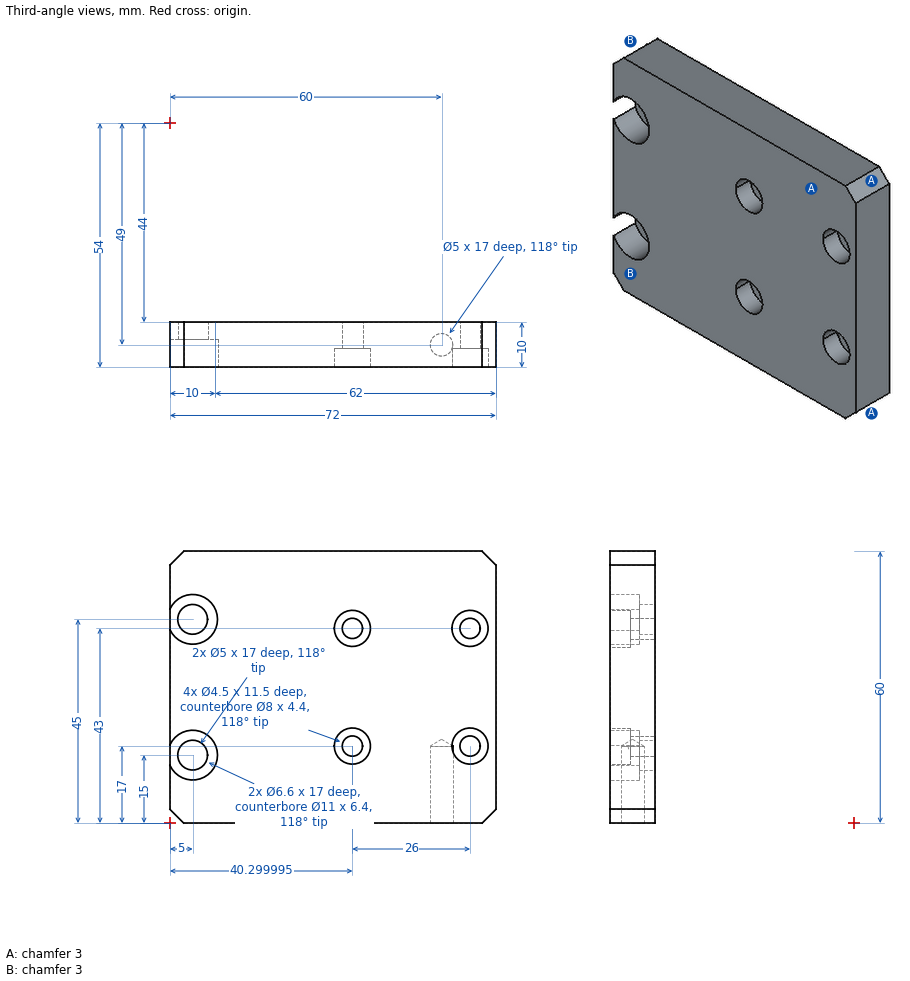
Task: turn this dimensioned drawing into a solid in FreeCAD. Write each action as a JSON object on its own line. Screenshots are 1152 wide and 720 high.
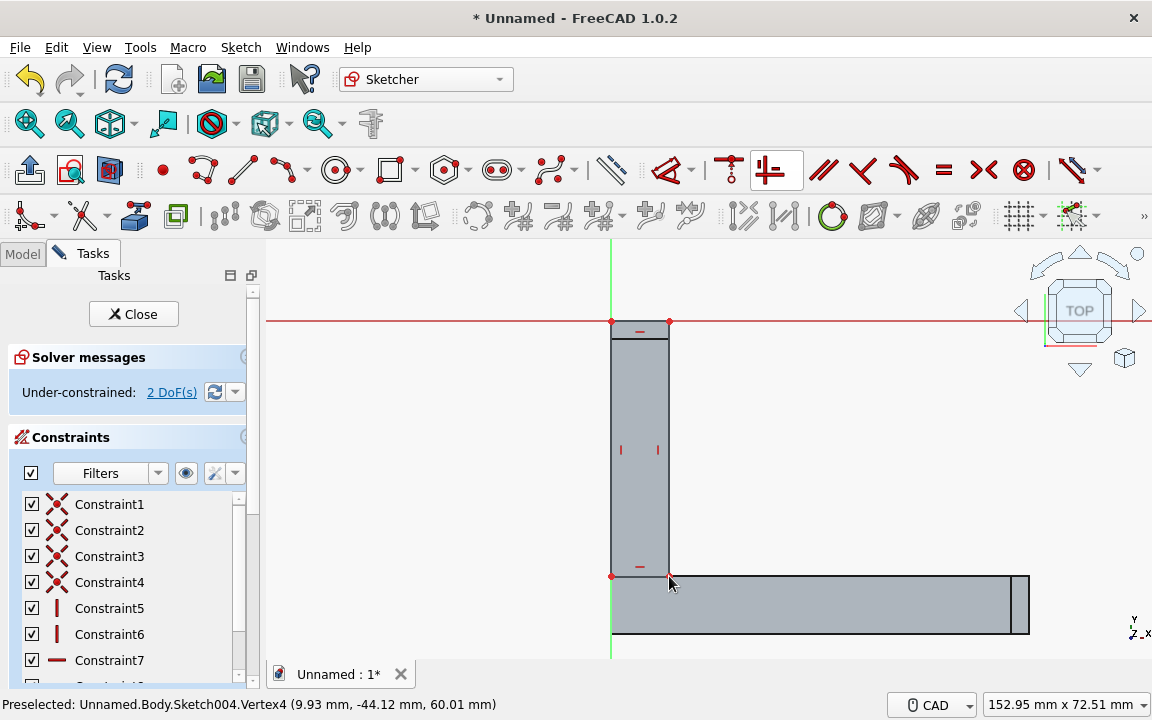
{"action": "left_click", "coordinate": [666, 170]}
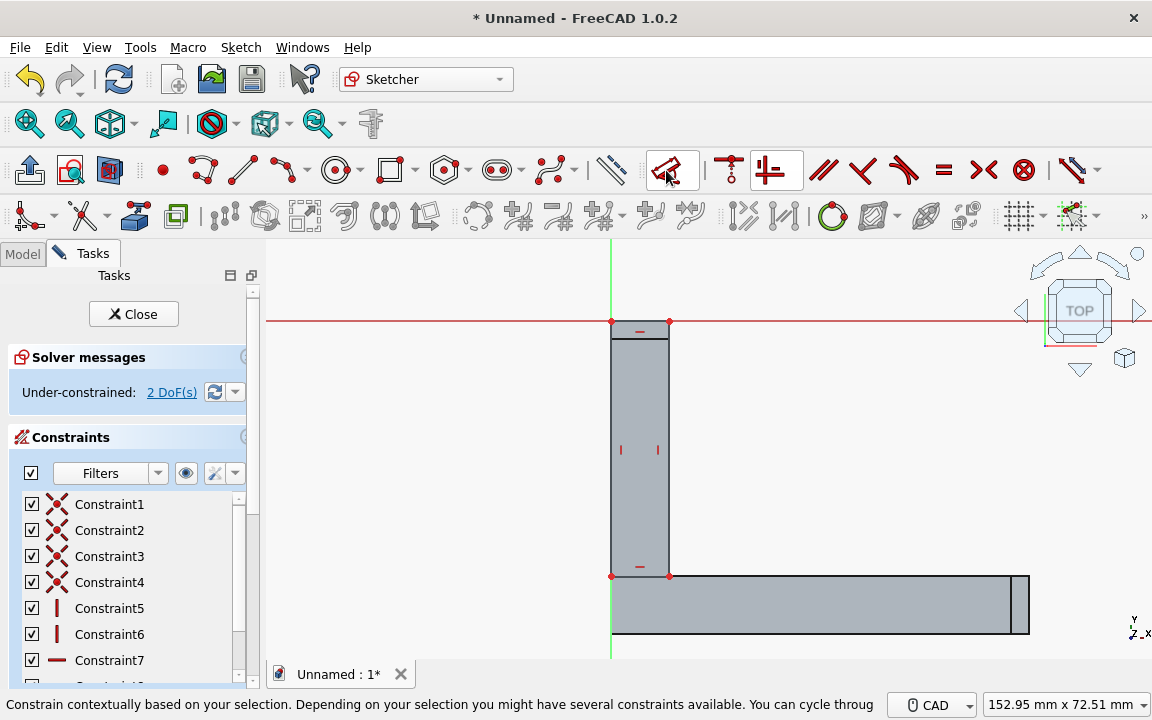
{"action": "left_click", "coordinate": [611, 398]}
{"action": "left_click", "coordinate": [577, 449]}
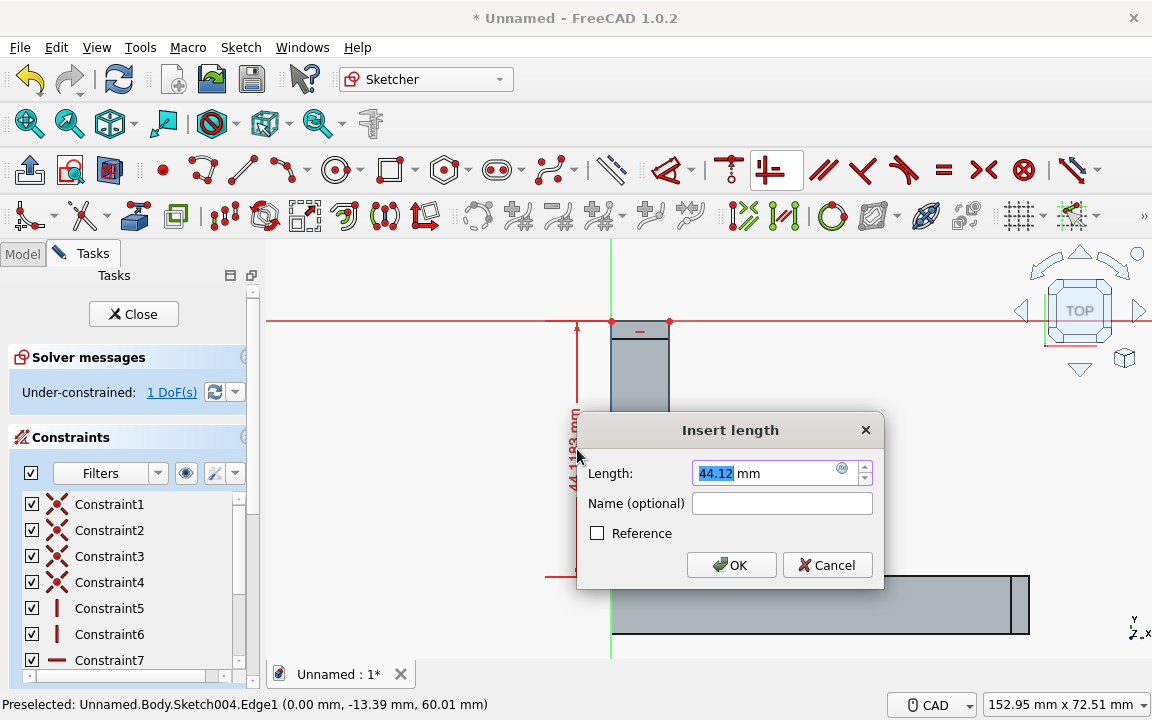
{"action": "type", "text": "44"}
{"action": "key", "text": "Return"}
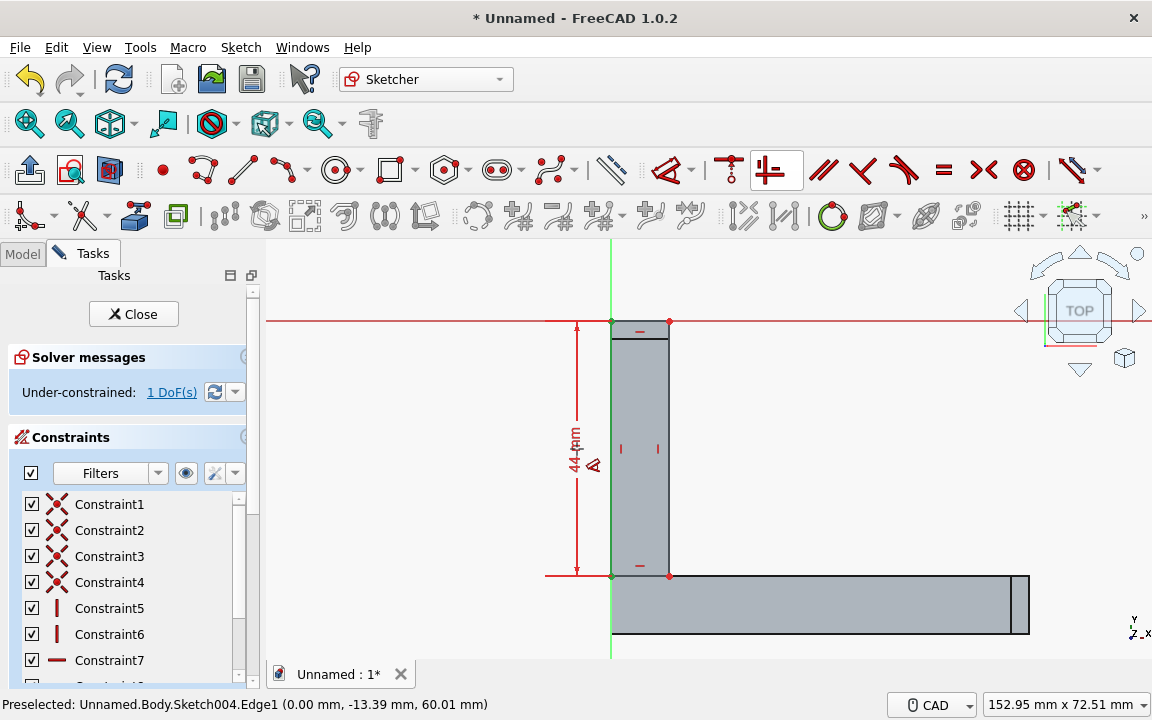
{"action": "left_click", "coordinate": [629, 576]}
{"action": "left_click", "coordinate": [640, 610]}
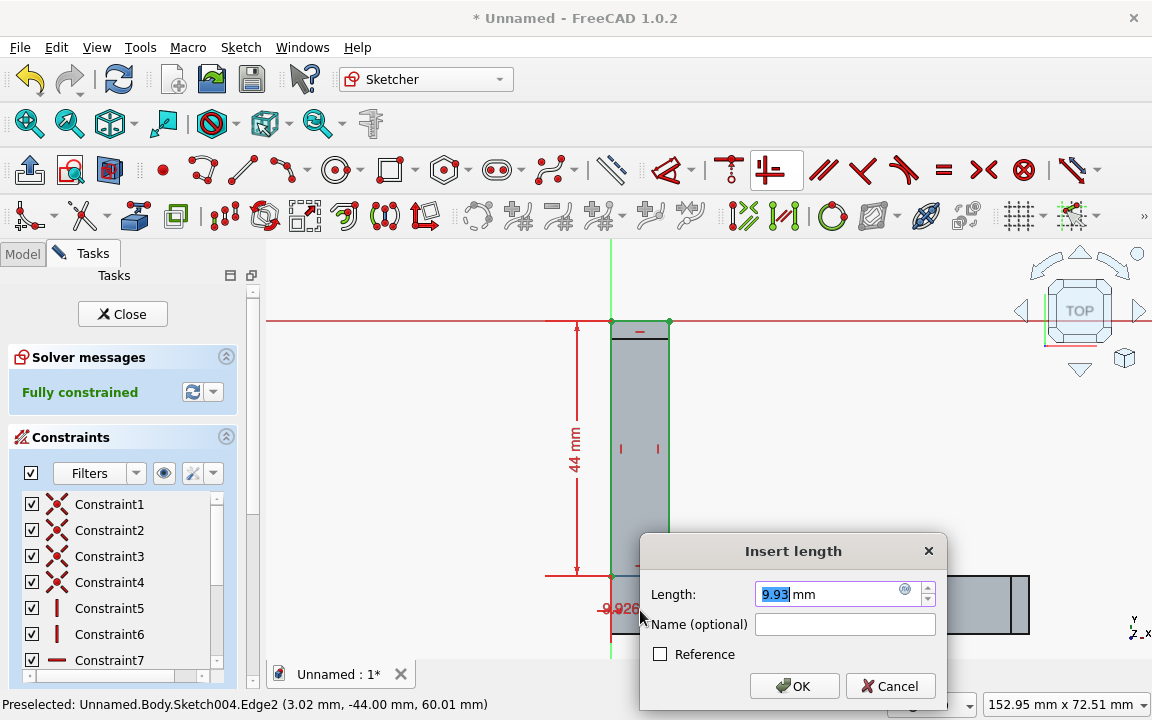
{"action": "type", "text": "10"}
{"action": "key", "text": "Return"}
{"action": "key", "text": "Escape"}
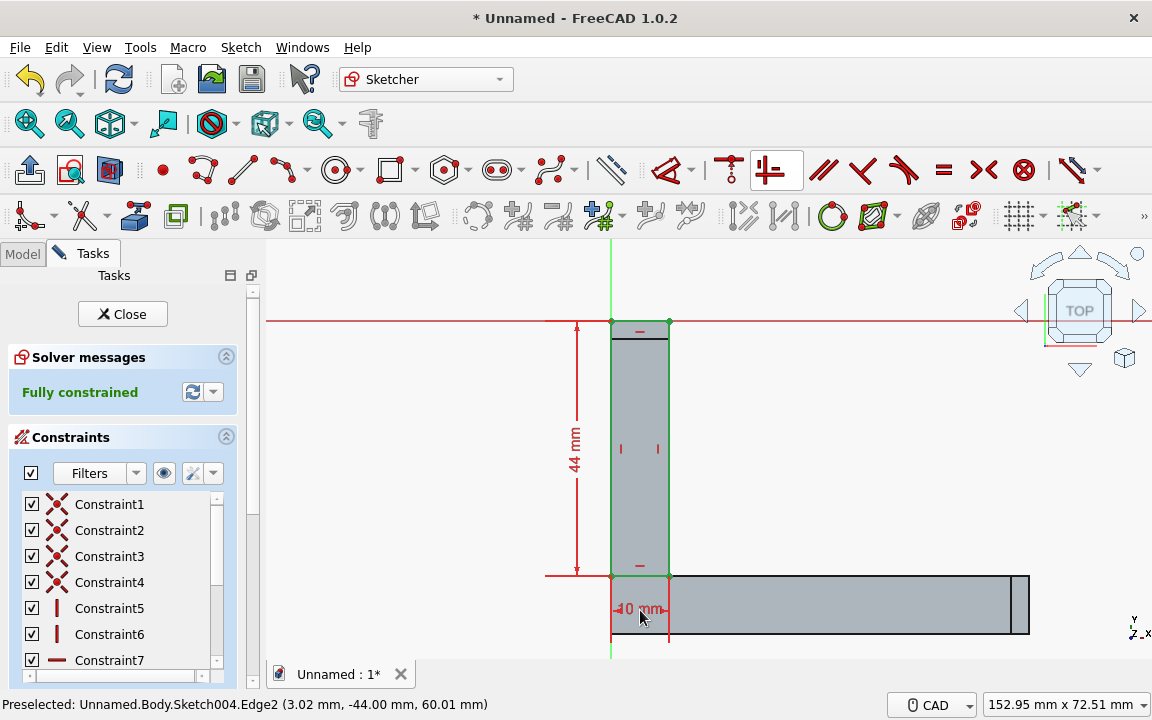
{"action": "left_click", "coordinate": [123, 314]}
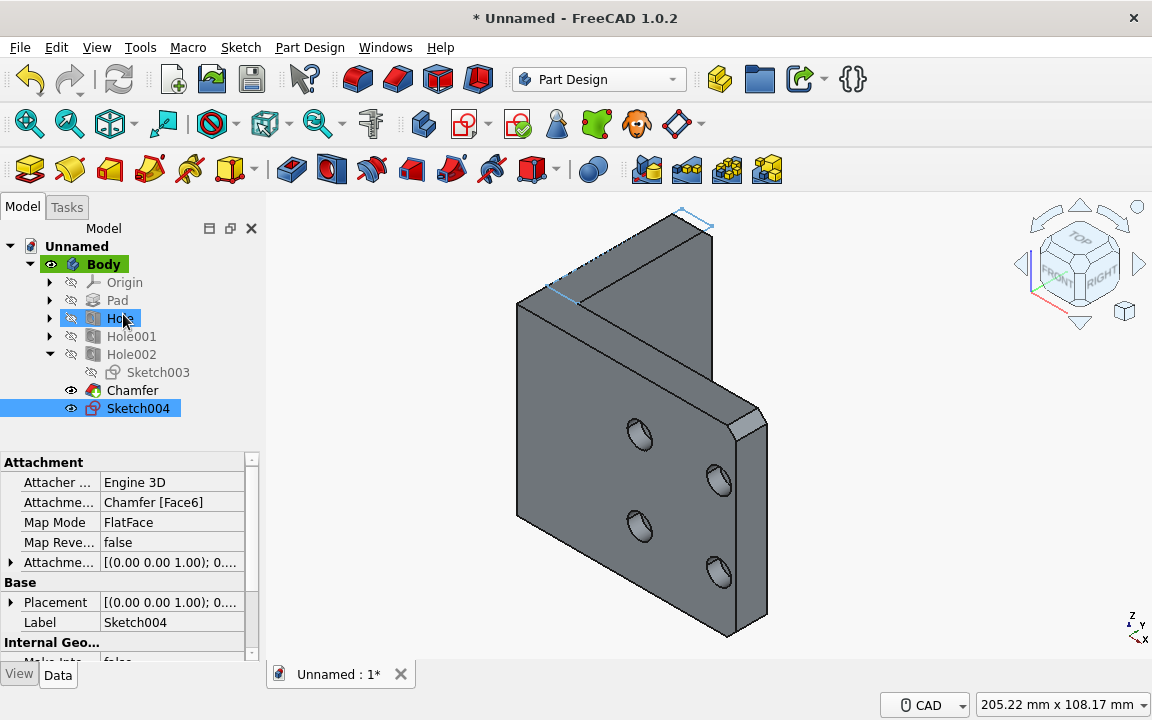
{"action": "left_click", "coordinate": [292, 170]}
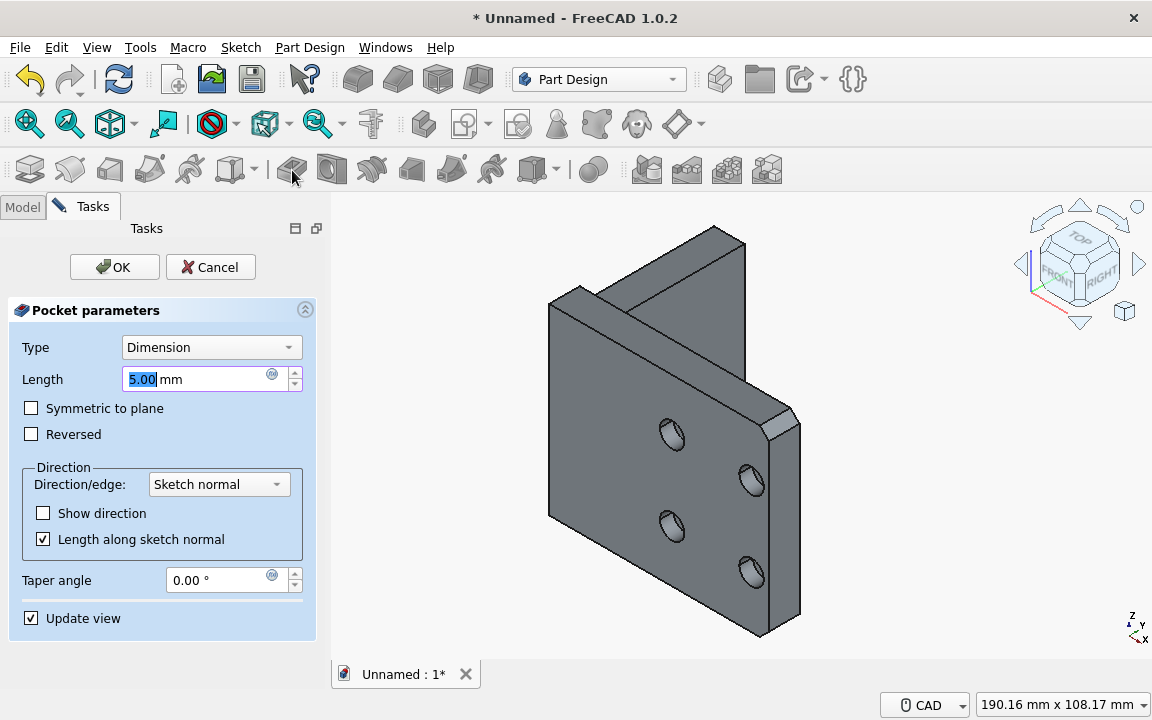
{"action": "left_click", "coordinate": [212, 348]}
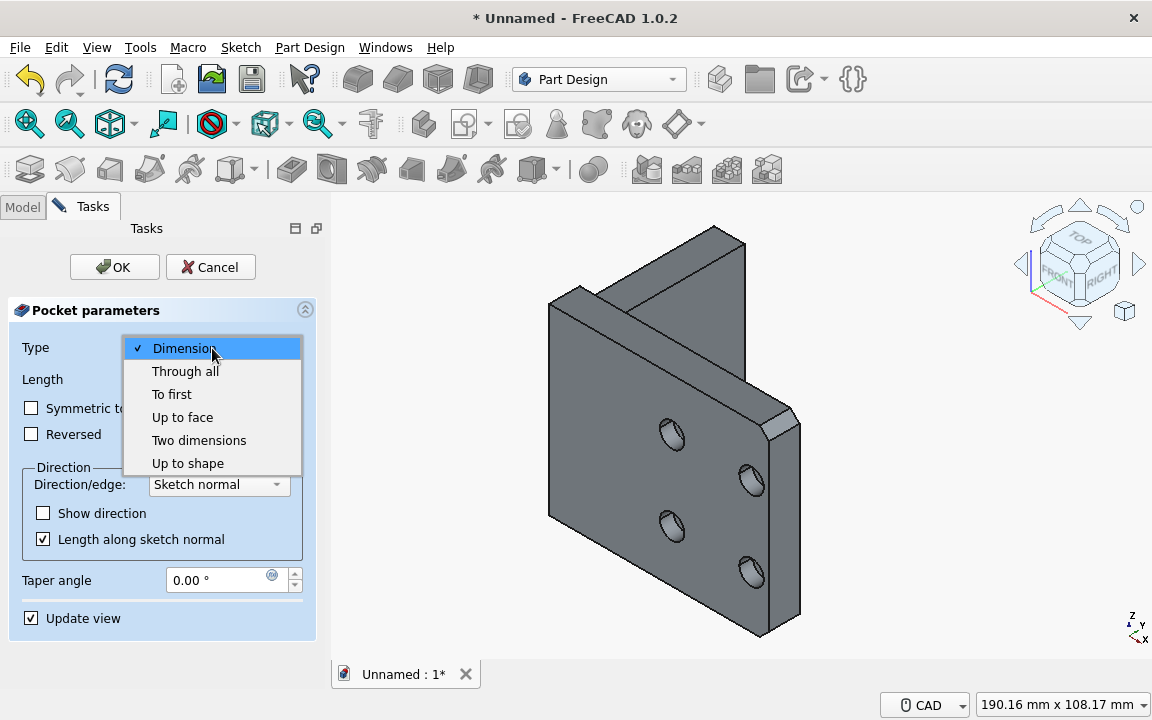
{"action": "left_click", "coordinate": [212, 372]}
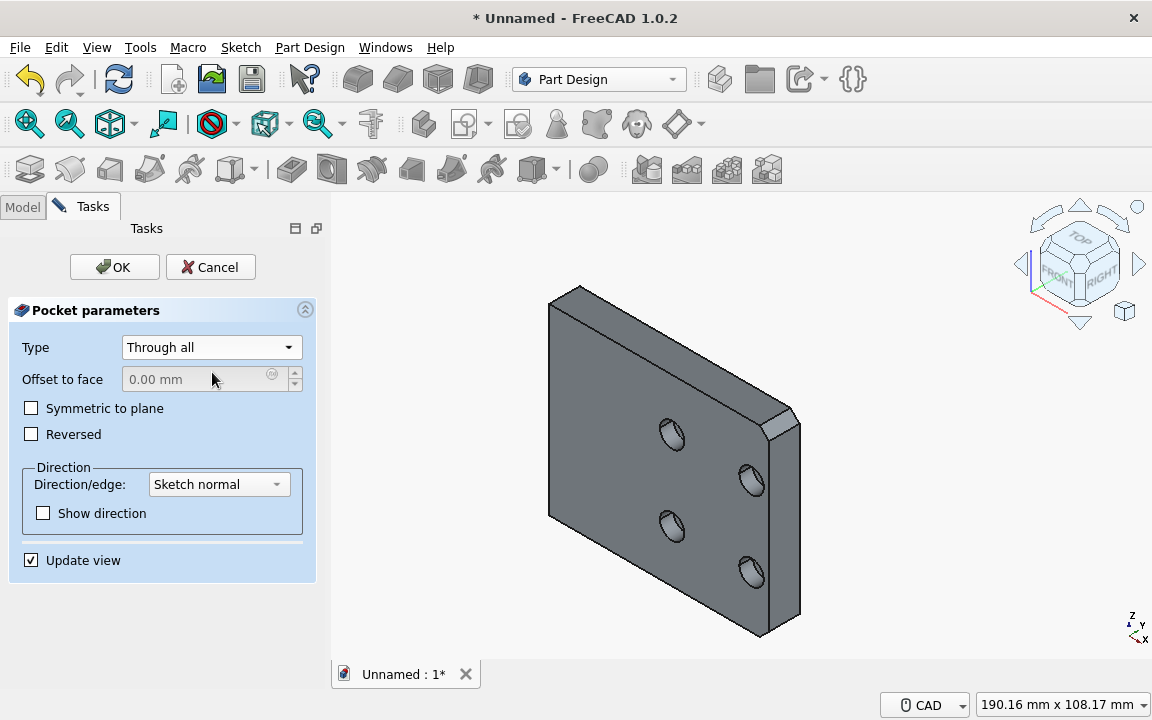
{"action": "left_click", "coordinate": [115, 267]}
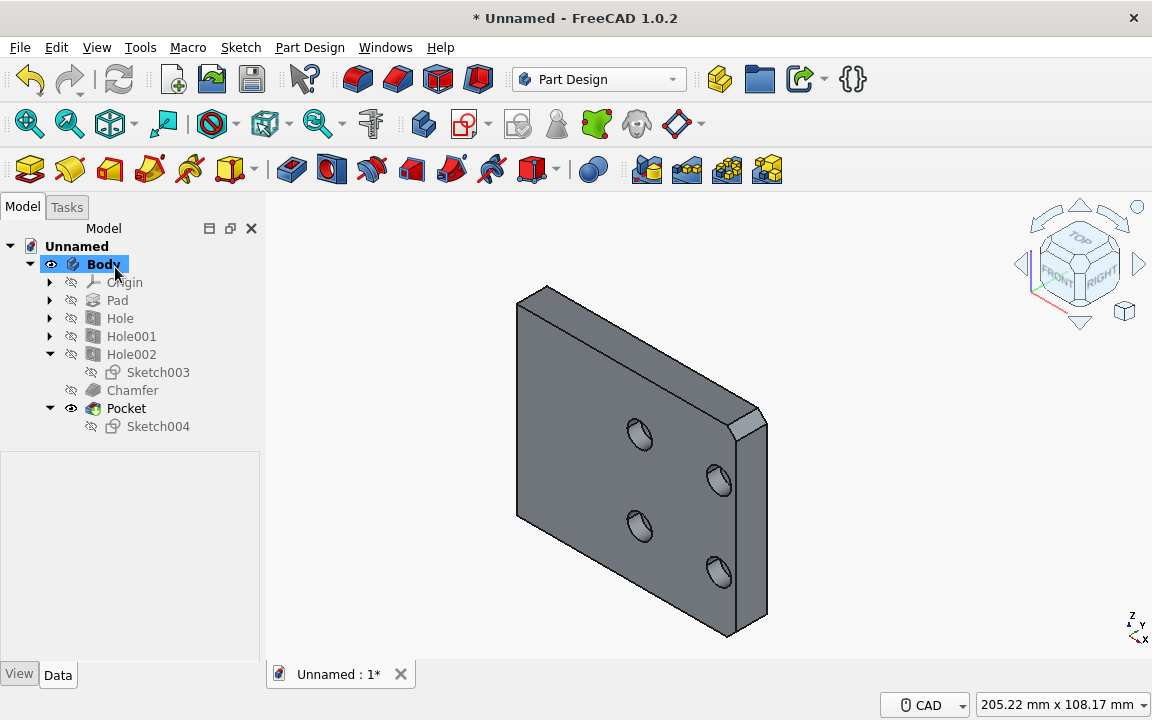
{"action": "key", "text": "2"}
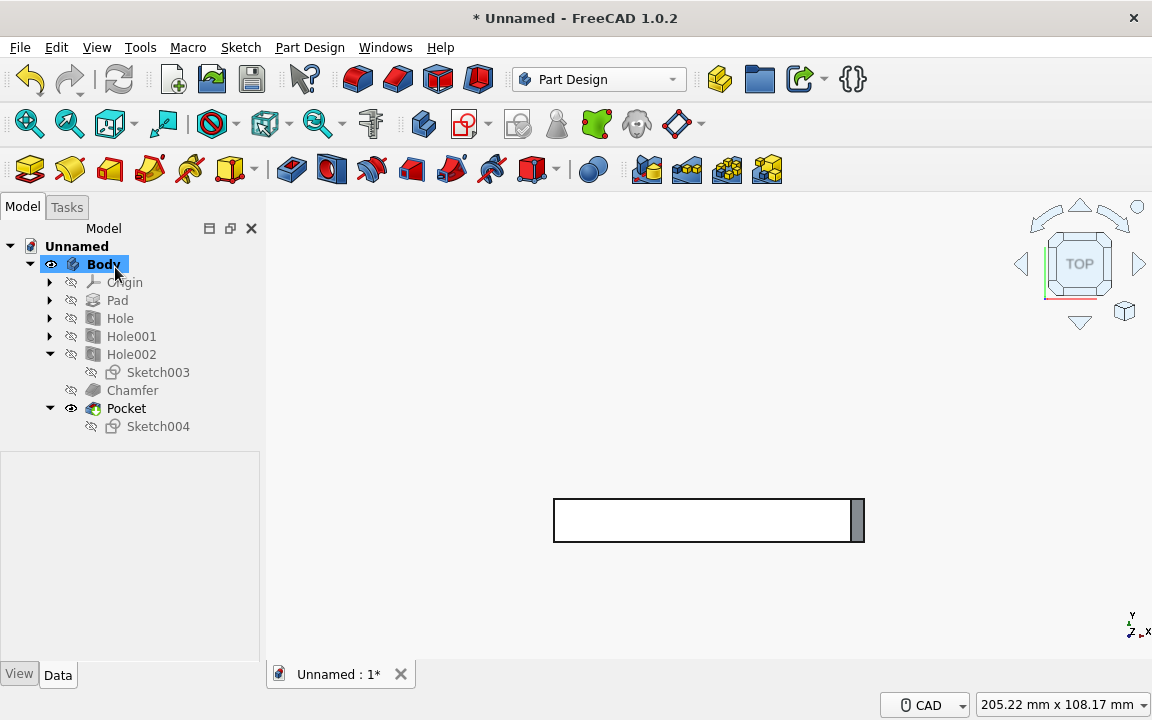
{"action": "left_click", "coordinate": [30, 124]}